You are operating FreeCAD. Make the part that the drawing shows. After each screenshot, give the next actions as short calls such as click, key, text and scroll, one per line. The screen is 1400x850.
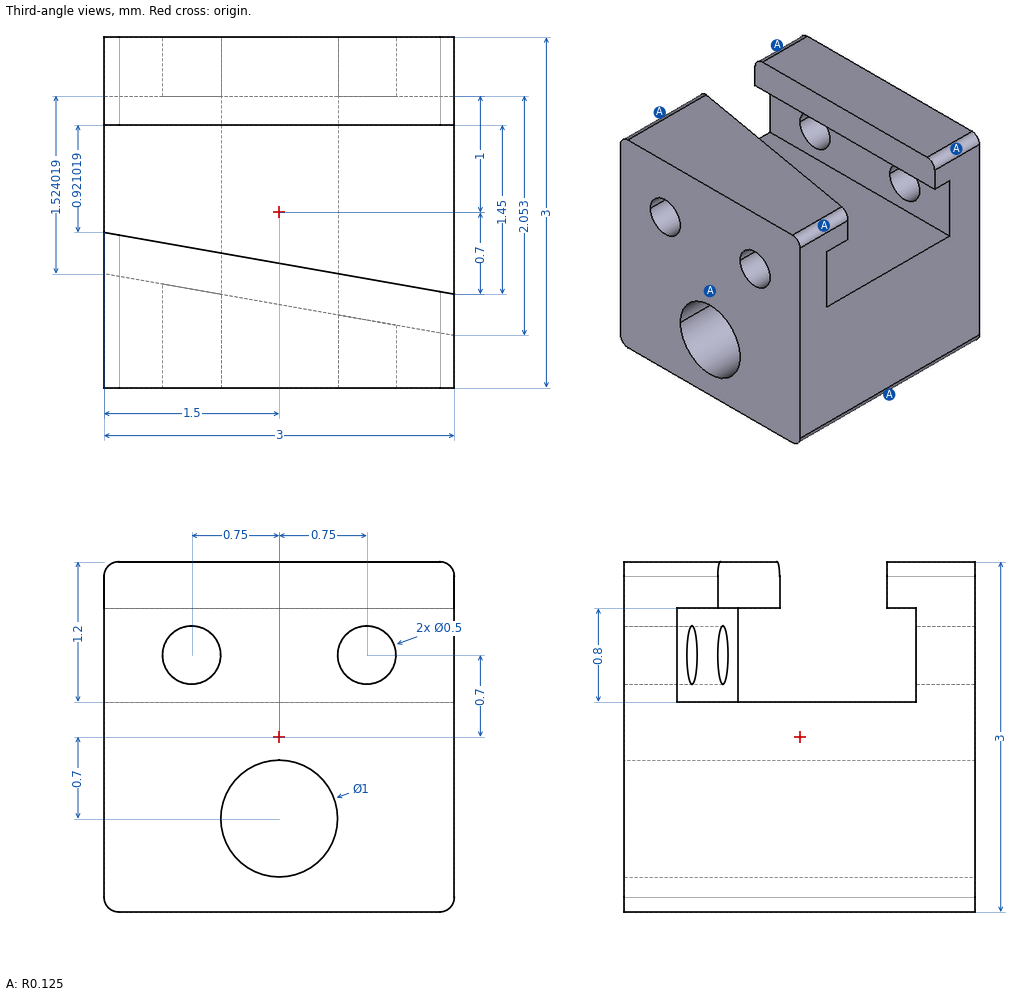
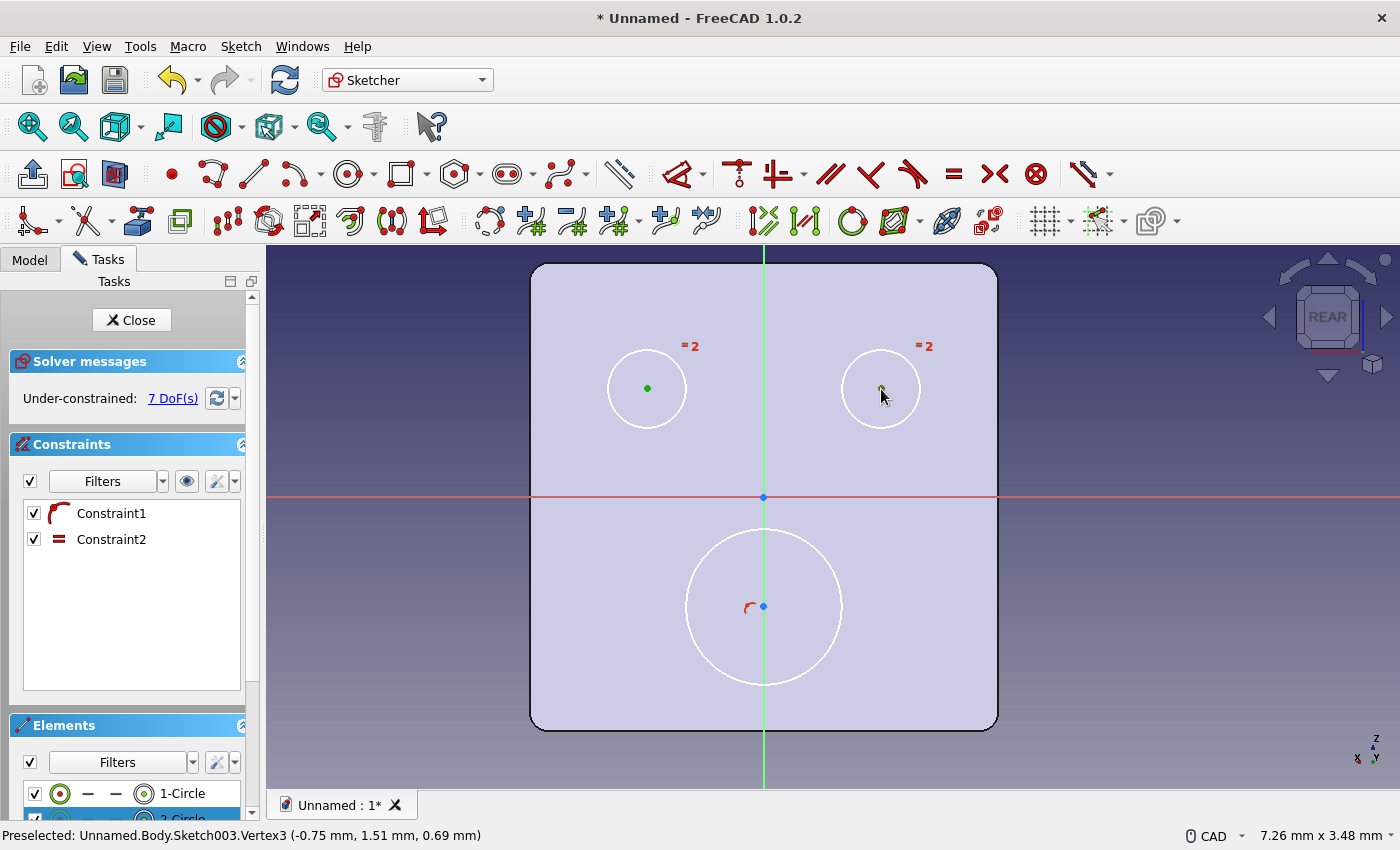
key(h)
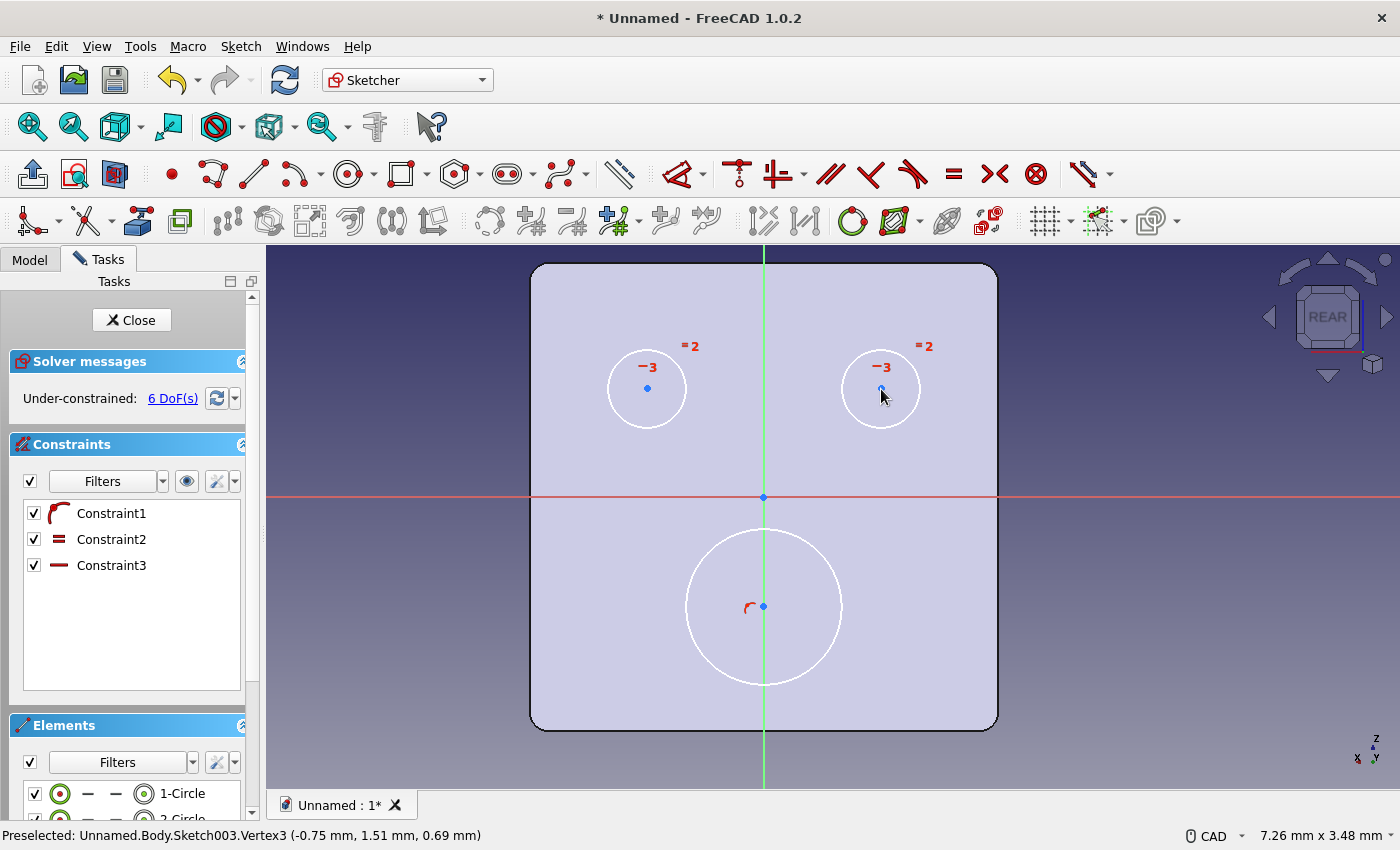
key(d)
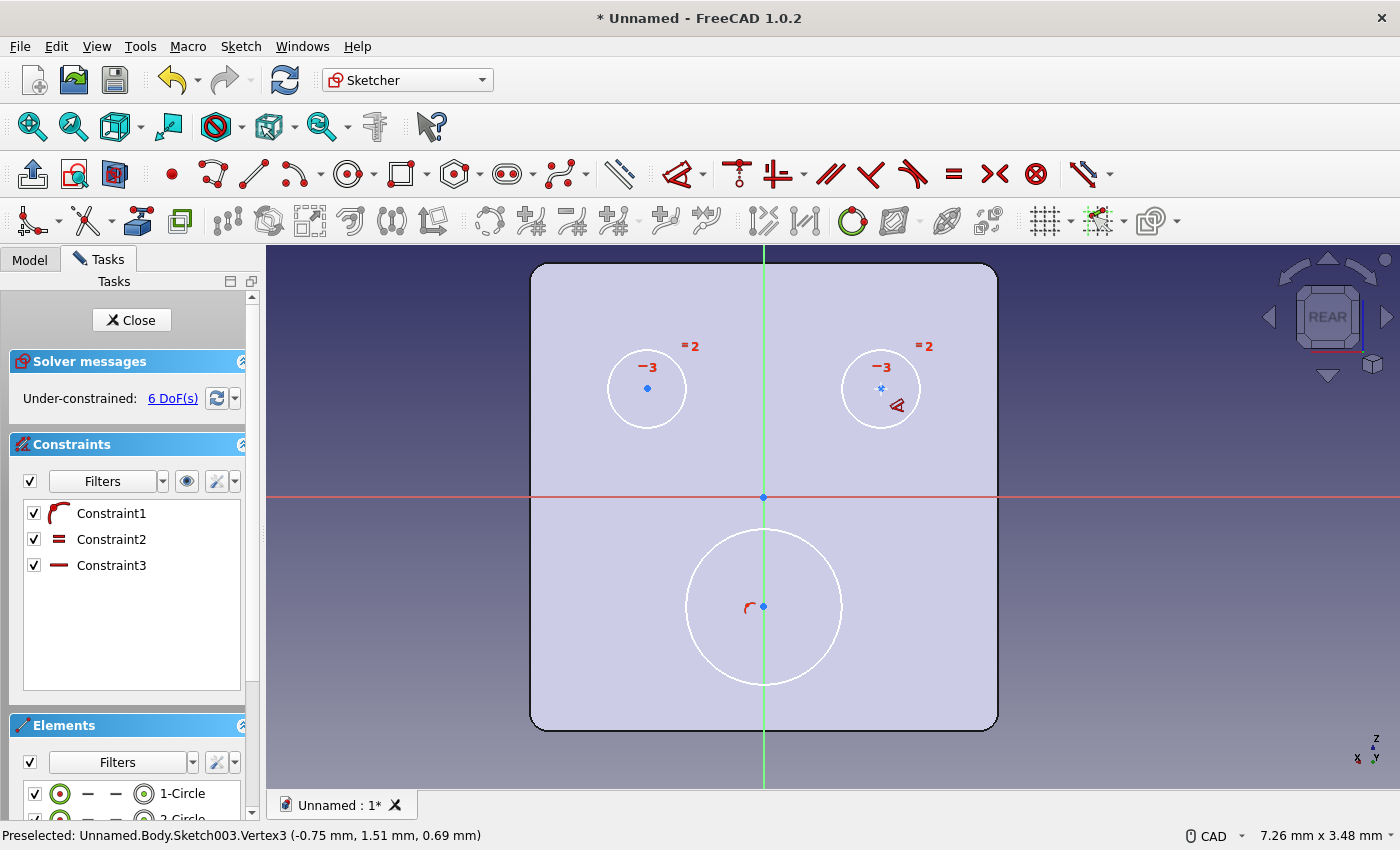
click(819, 552)
click(842, 529)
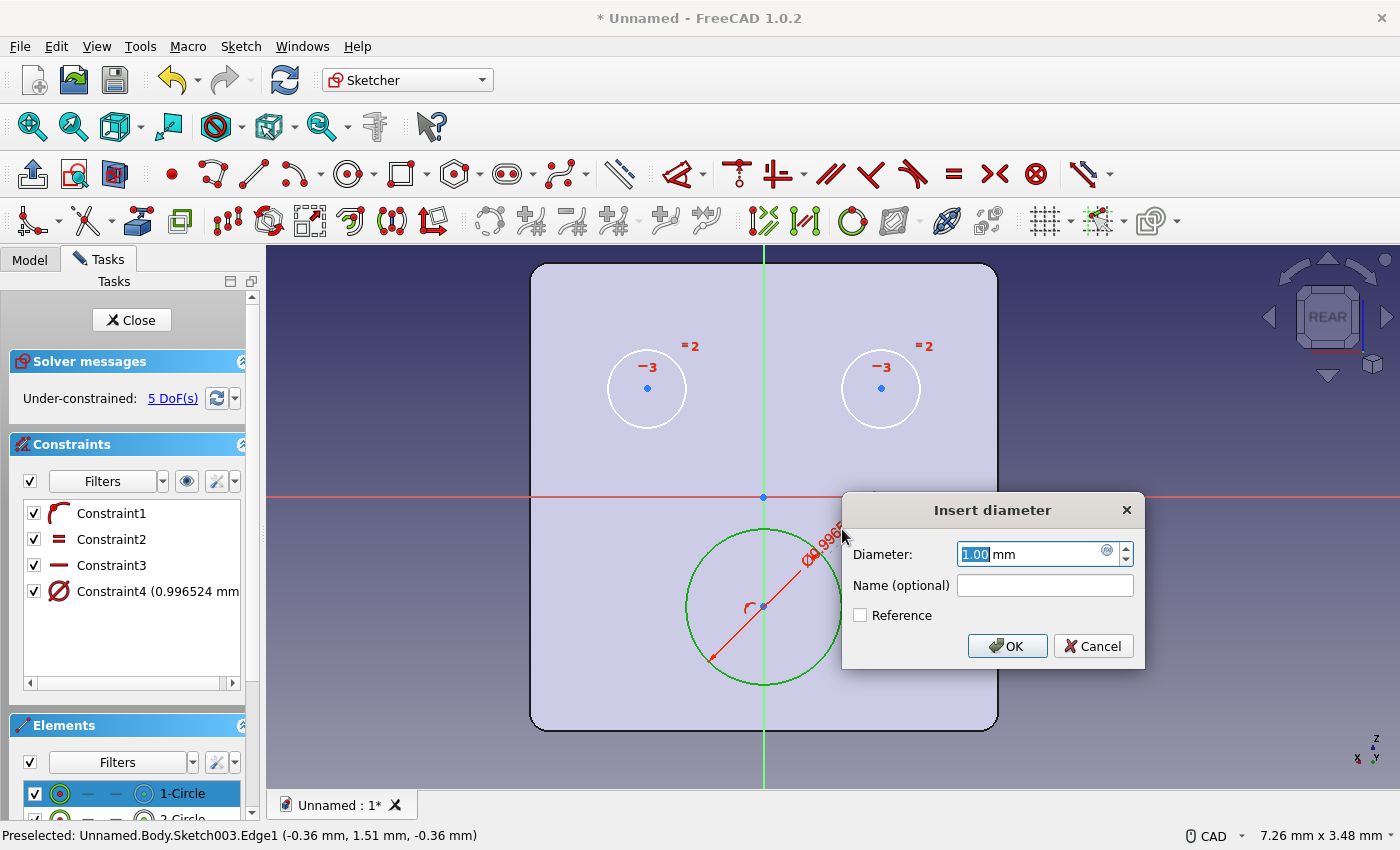
text(1)
key(Return)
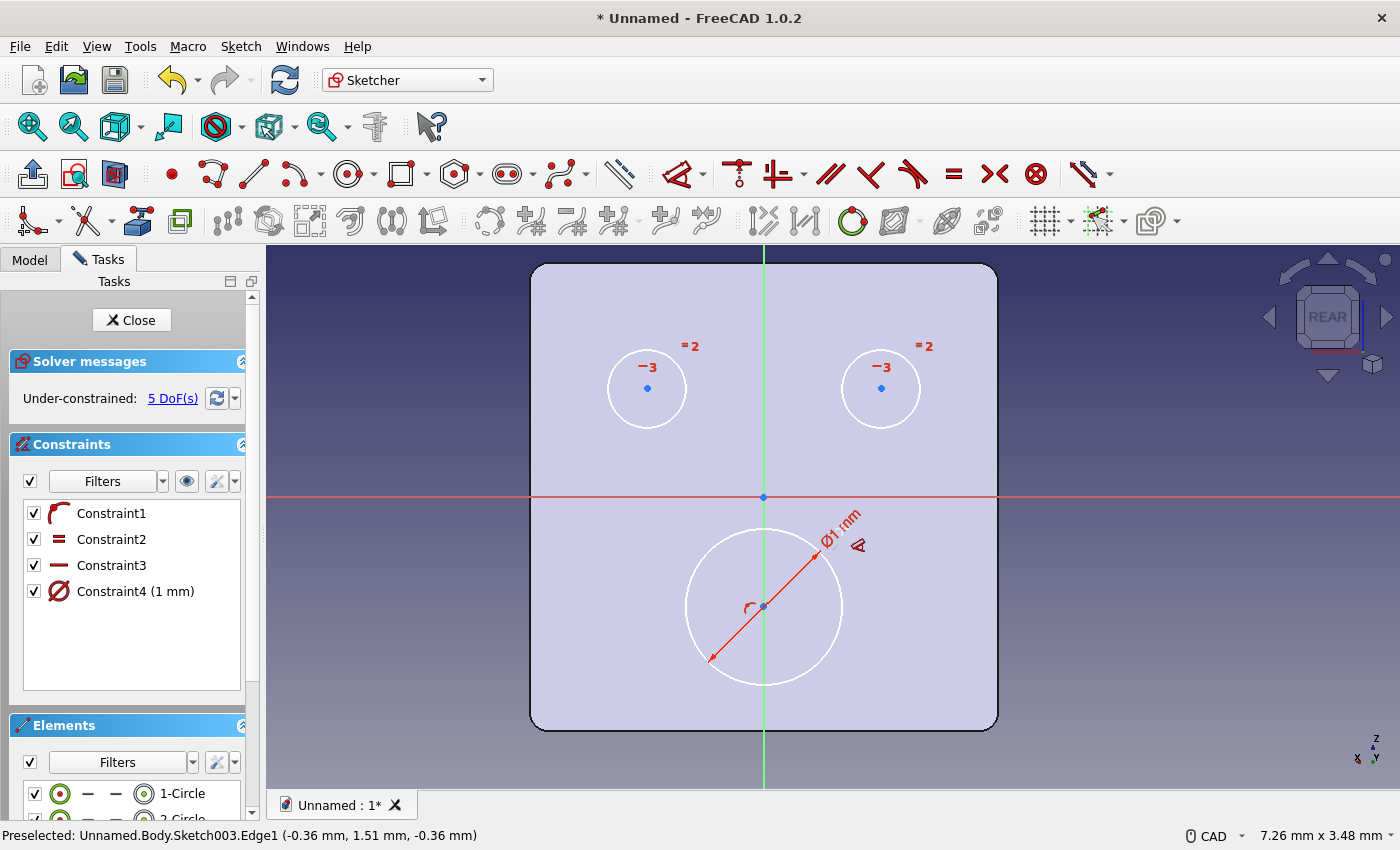
click(674, 361)
click(696, 338)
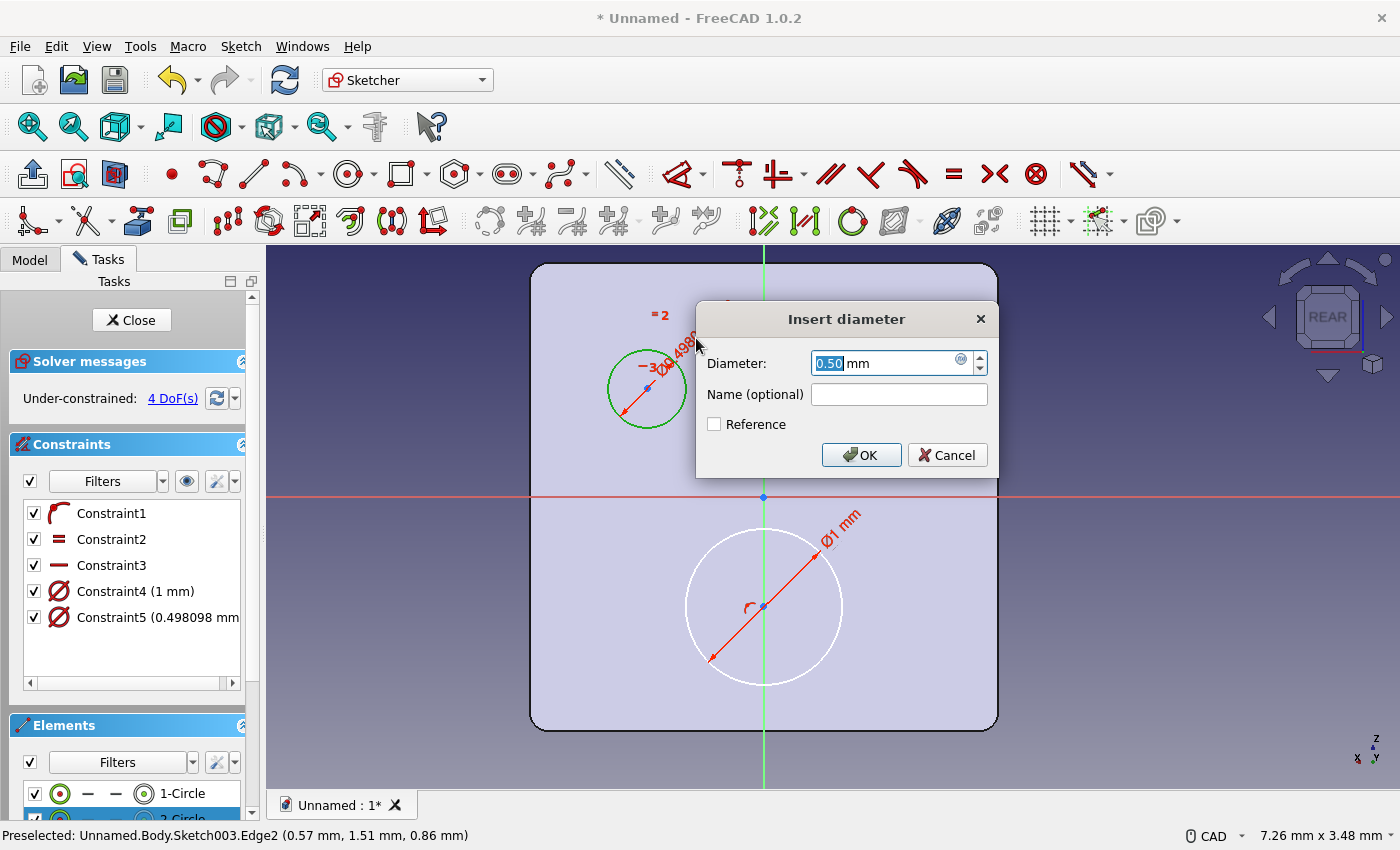
text(0.5)
key(Return)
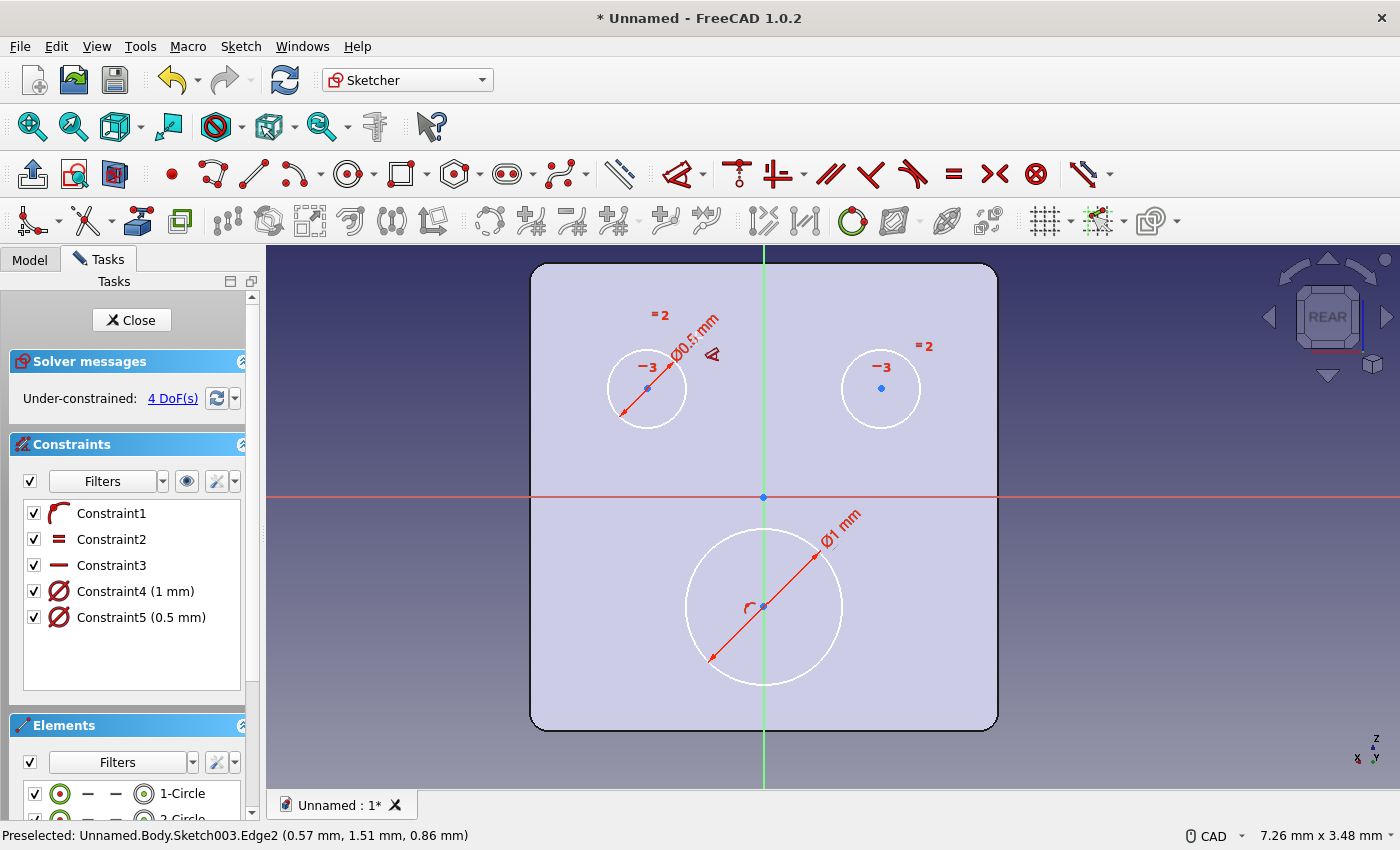
click(764, 607)
click(798, 552)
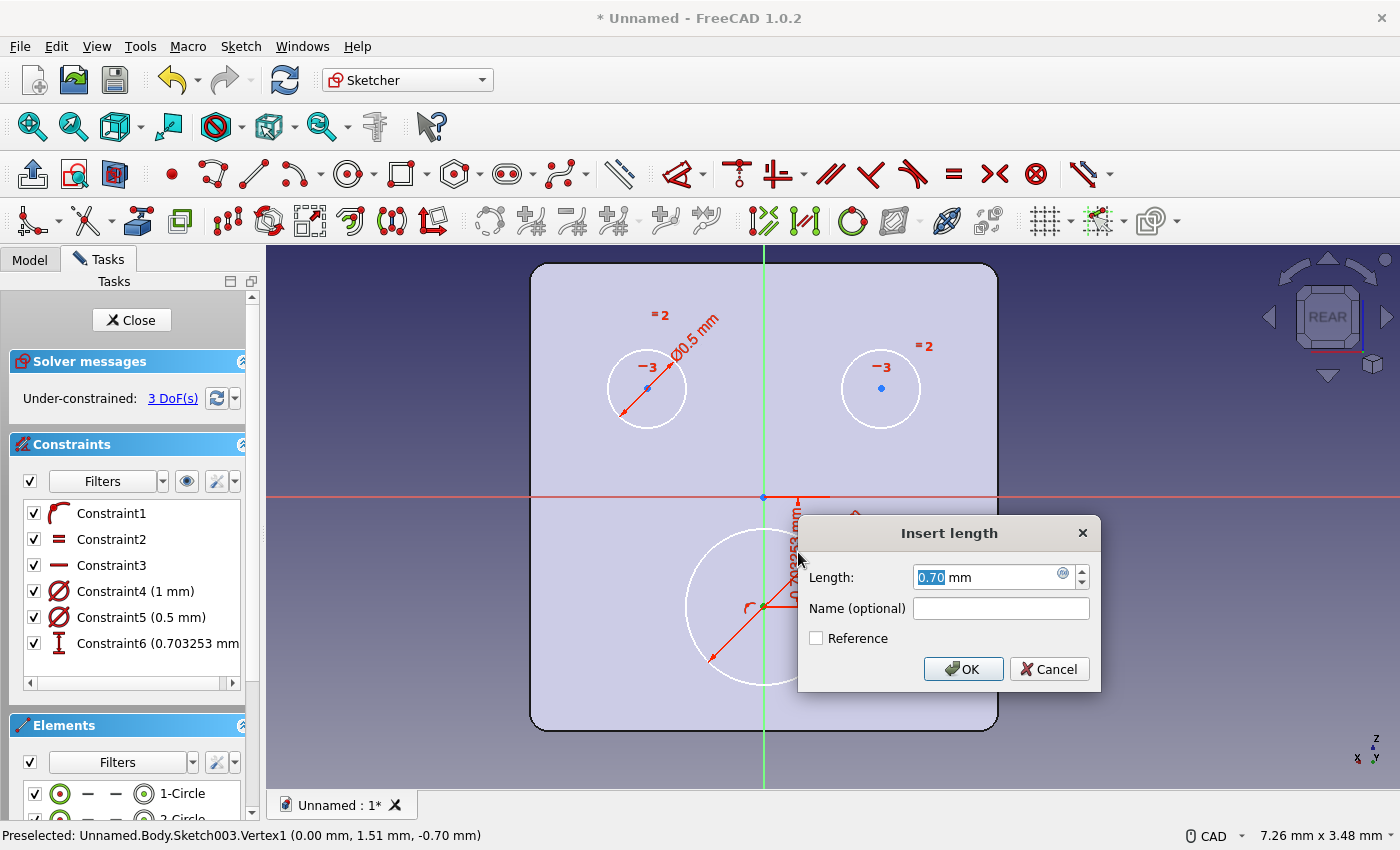
text(0.7)
key(Return)